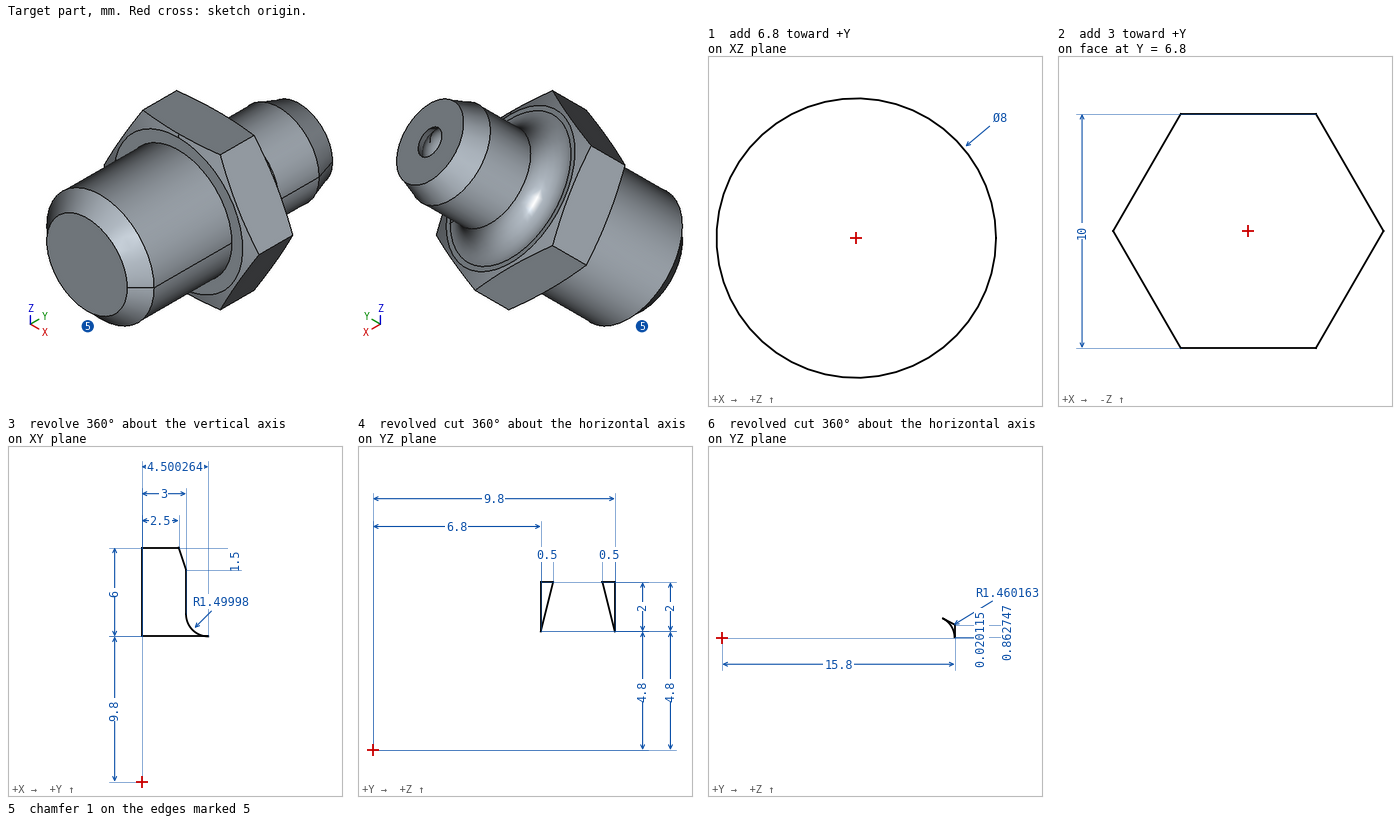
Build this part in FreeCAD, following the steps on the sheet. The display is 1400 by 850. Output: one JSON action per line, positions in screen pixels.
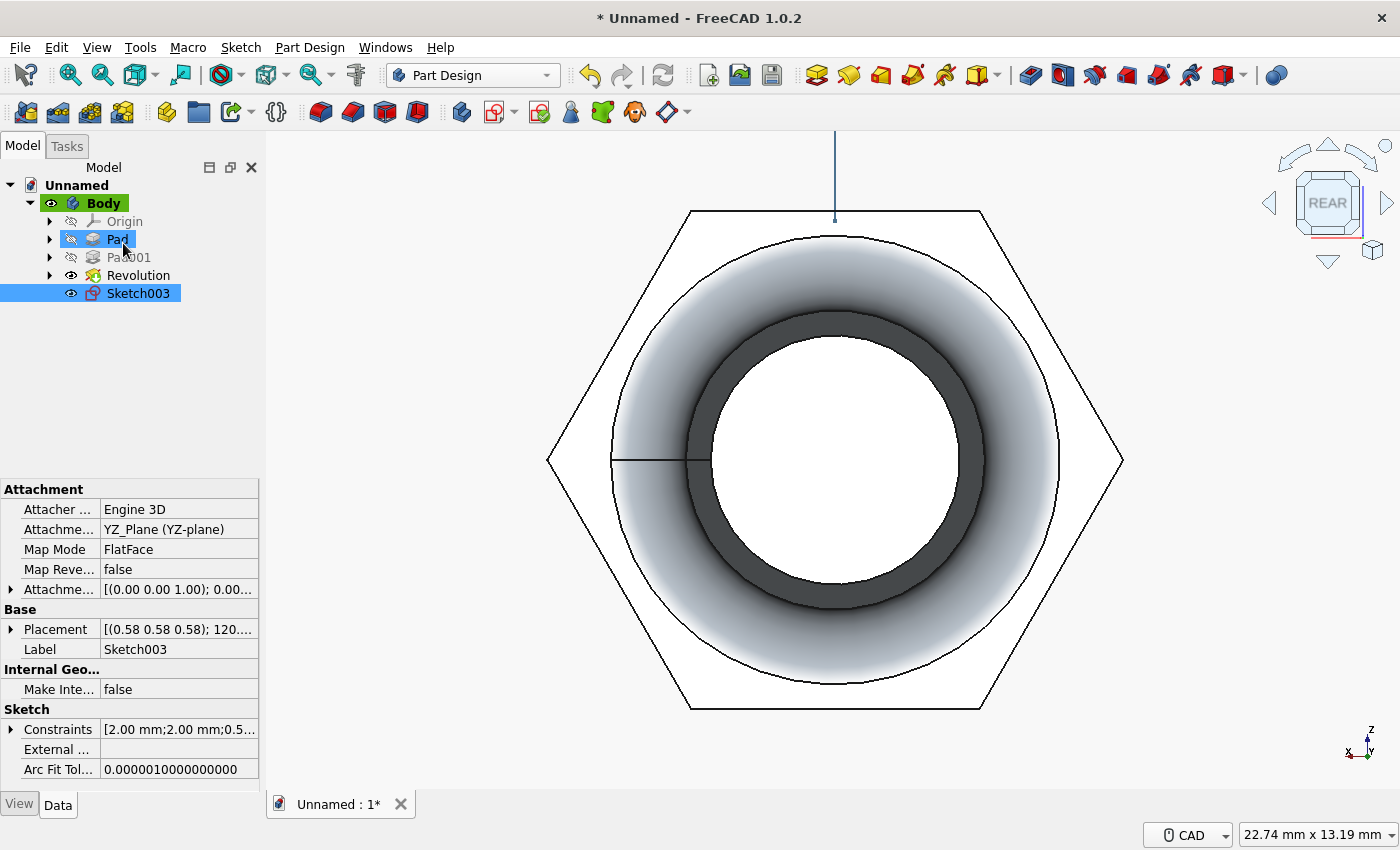
{"action": "left_click", "coordinate": [1096, 76]}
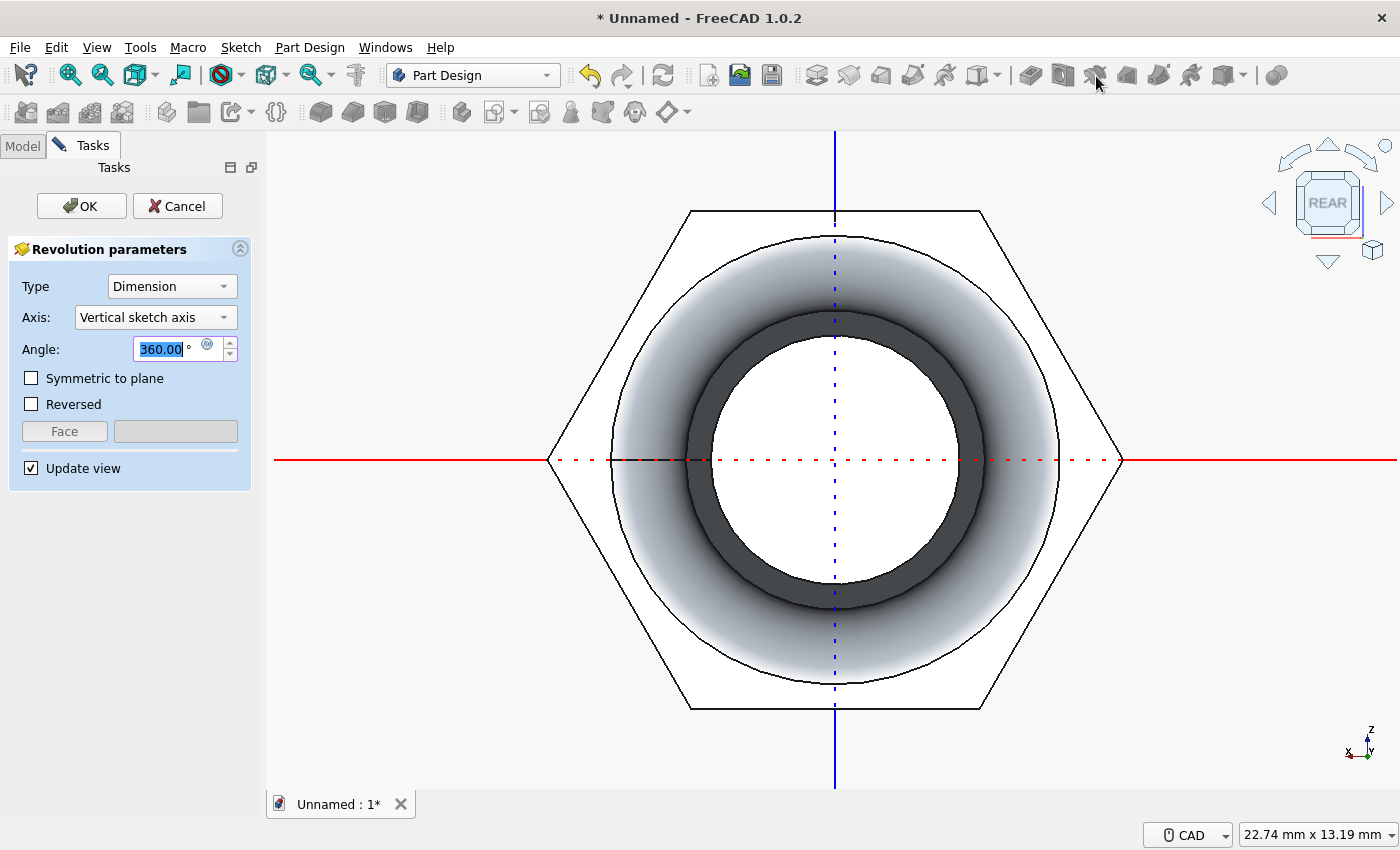
{"action": "left_click", "coordinate": [156, 318]}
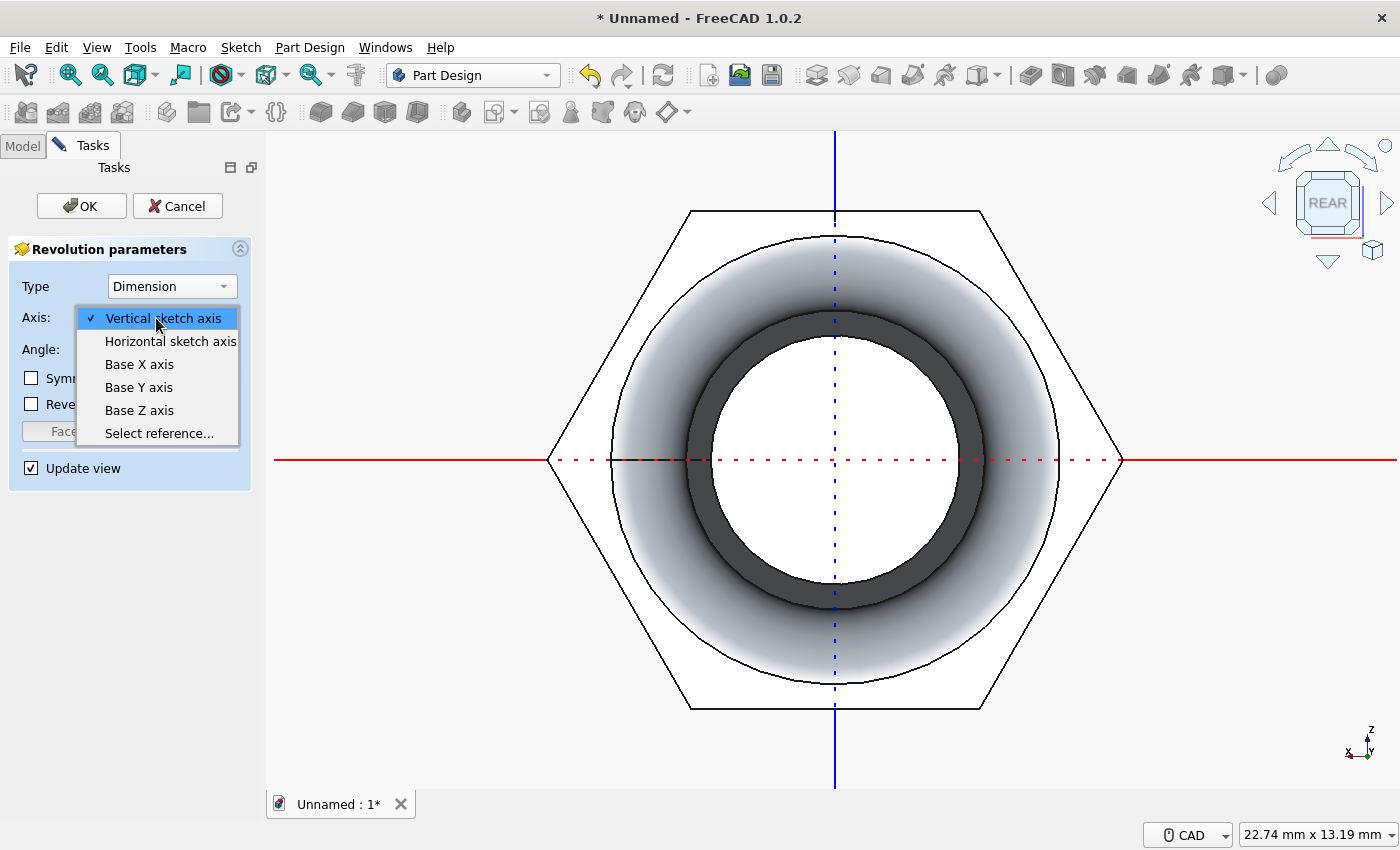
{"action": "left_click", "coordinate": [156, 342]}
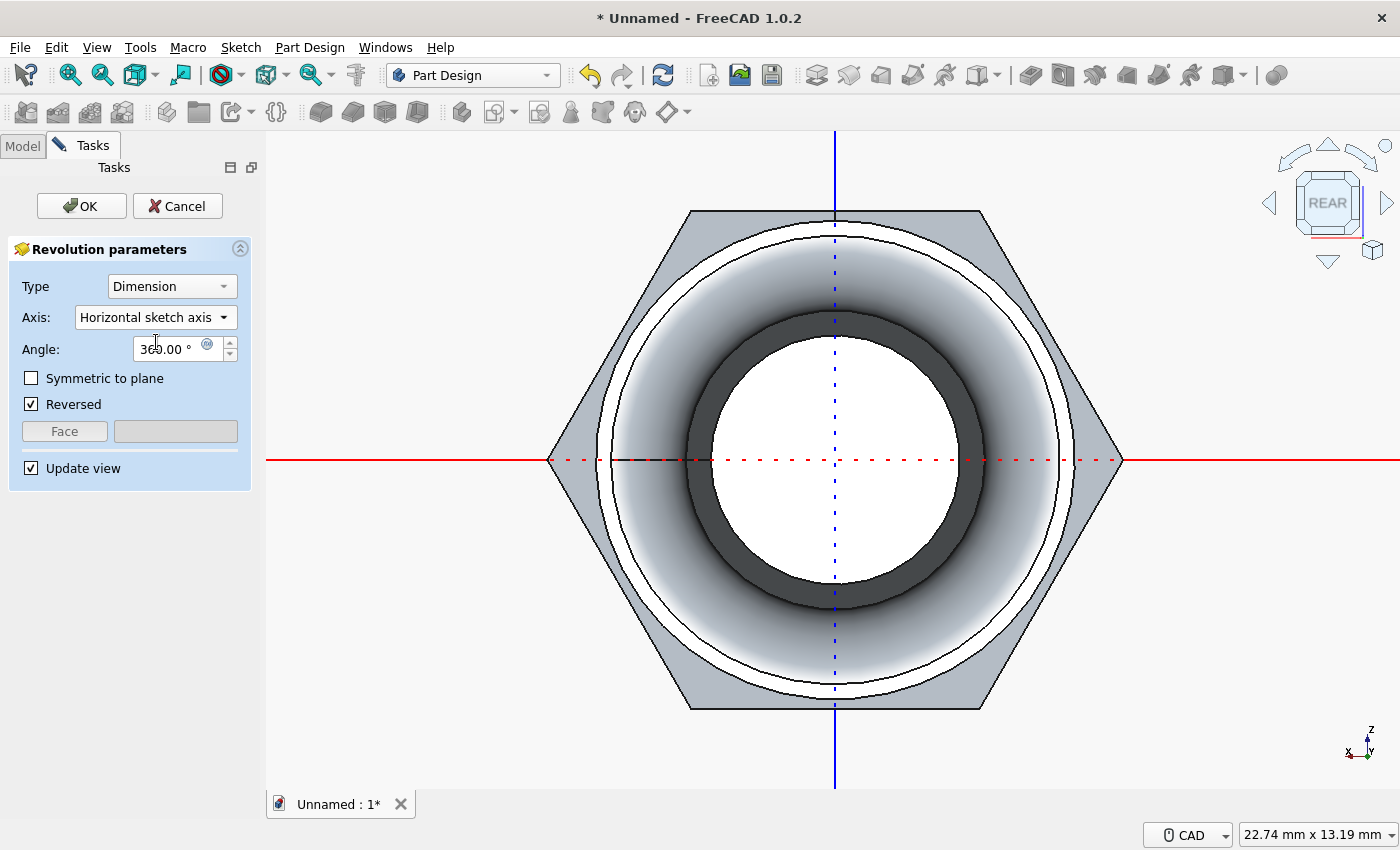
{"action": "left_click", "coordinate": [82, 206]}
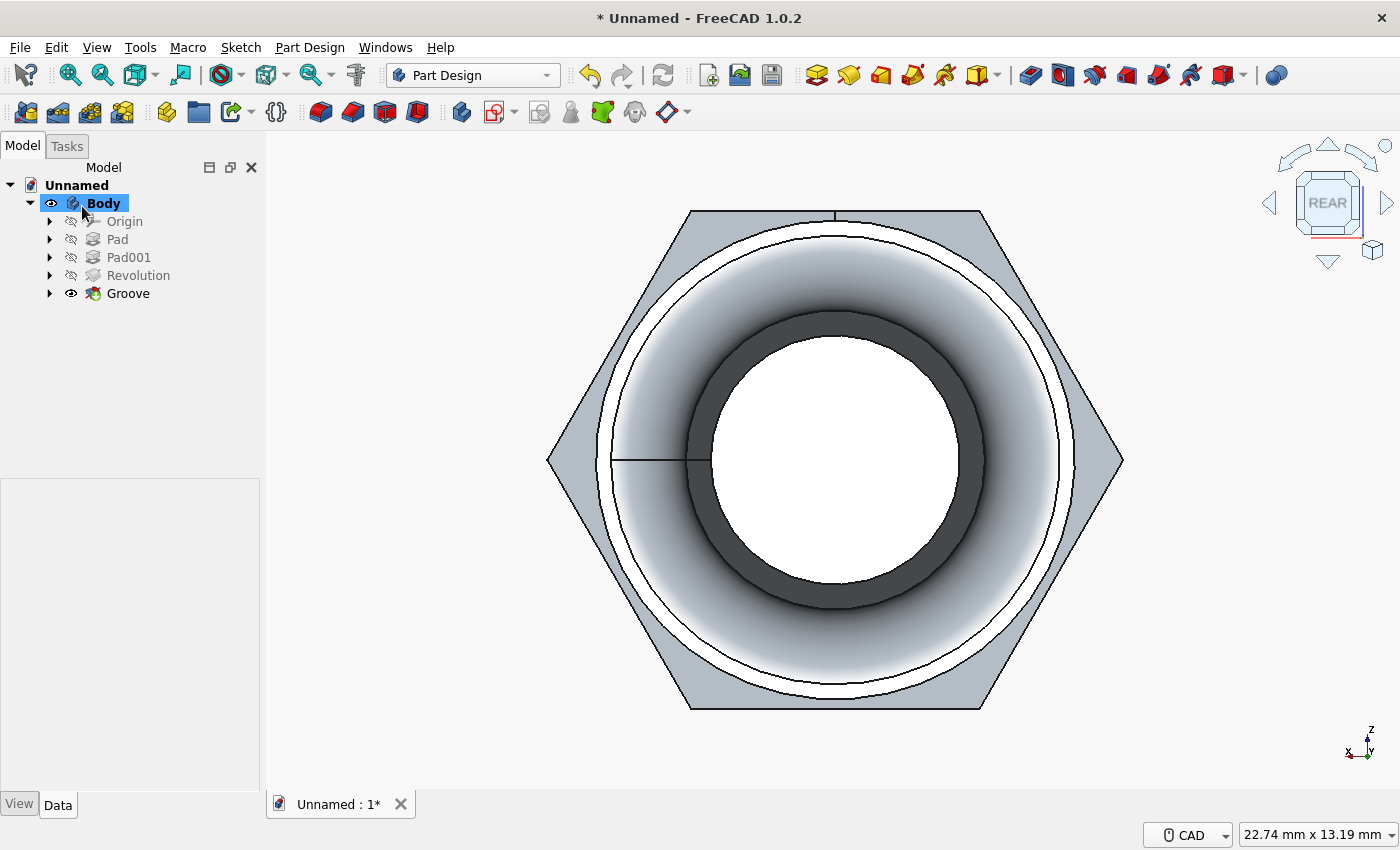
{"action": "key", "text": "0"}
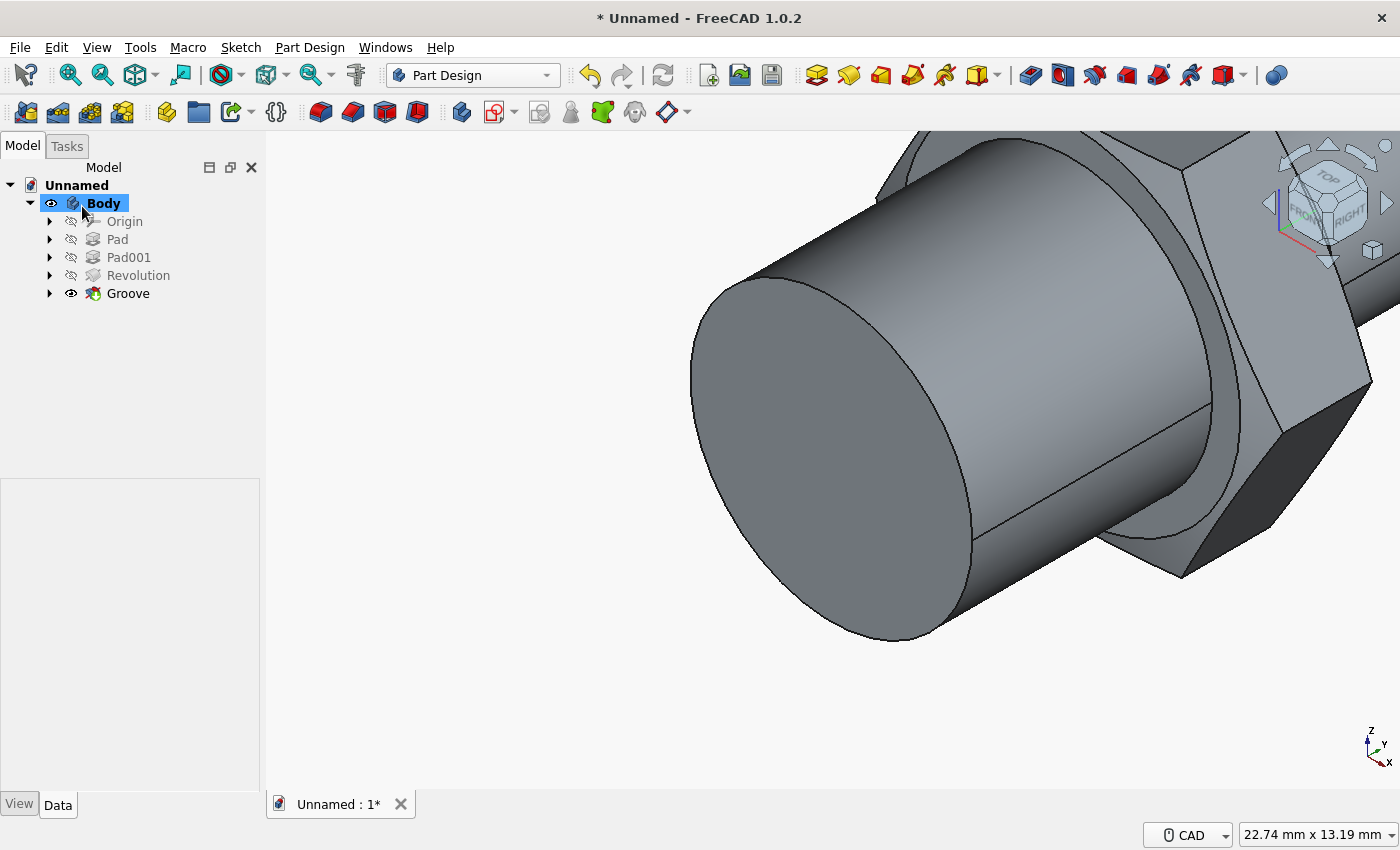
{"action": "left_click", "coordinate": [72, 76]}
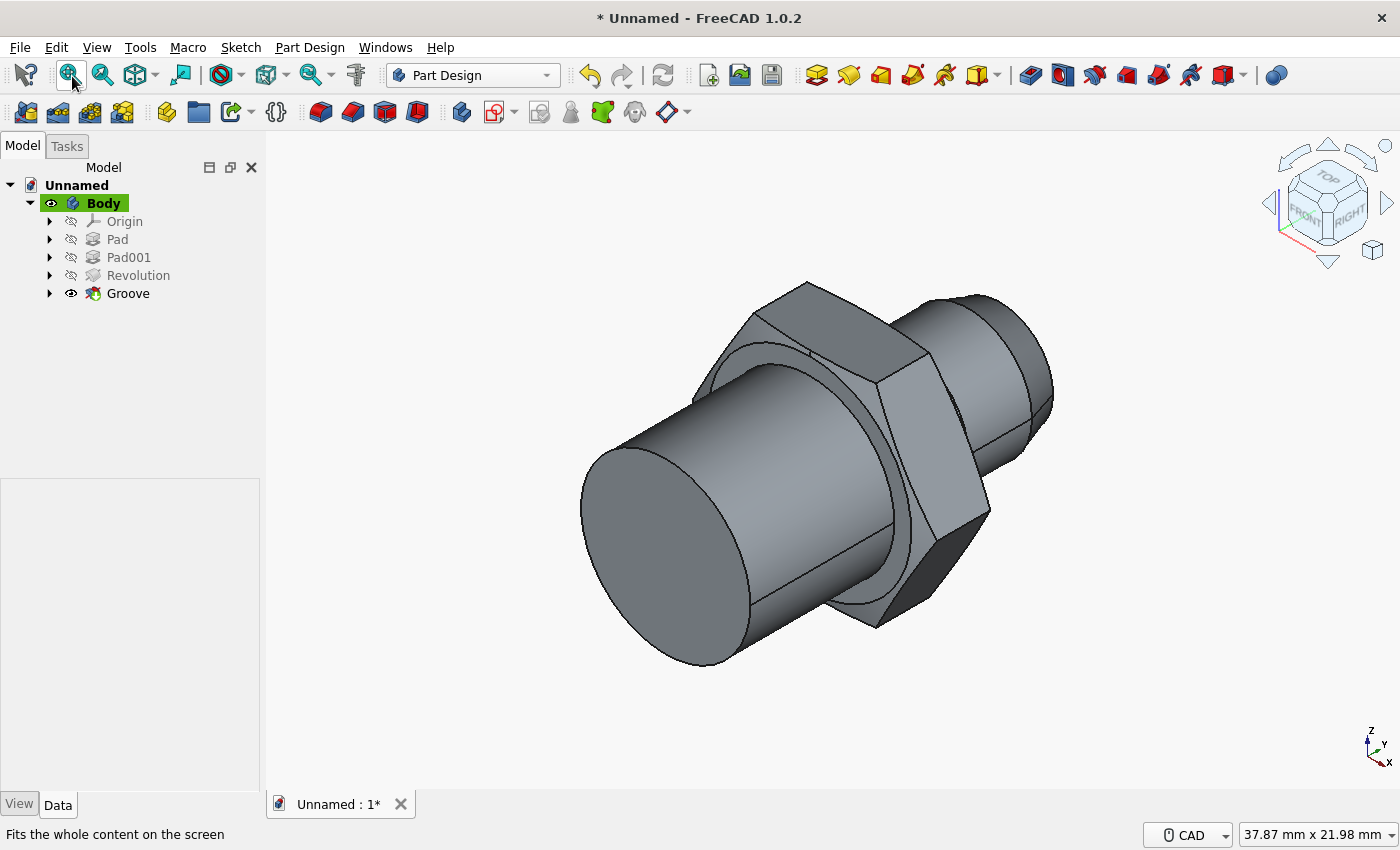
{"action": "left_click", "coordinate": [640, 447]}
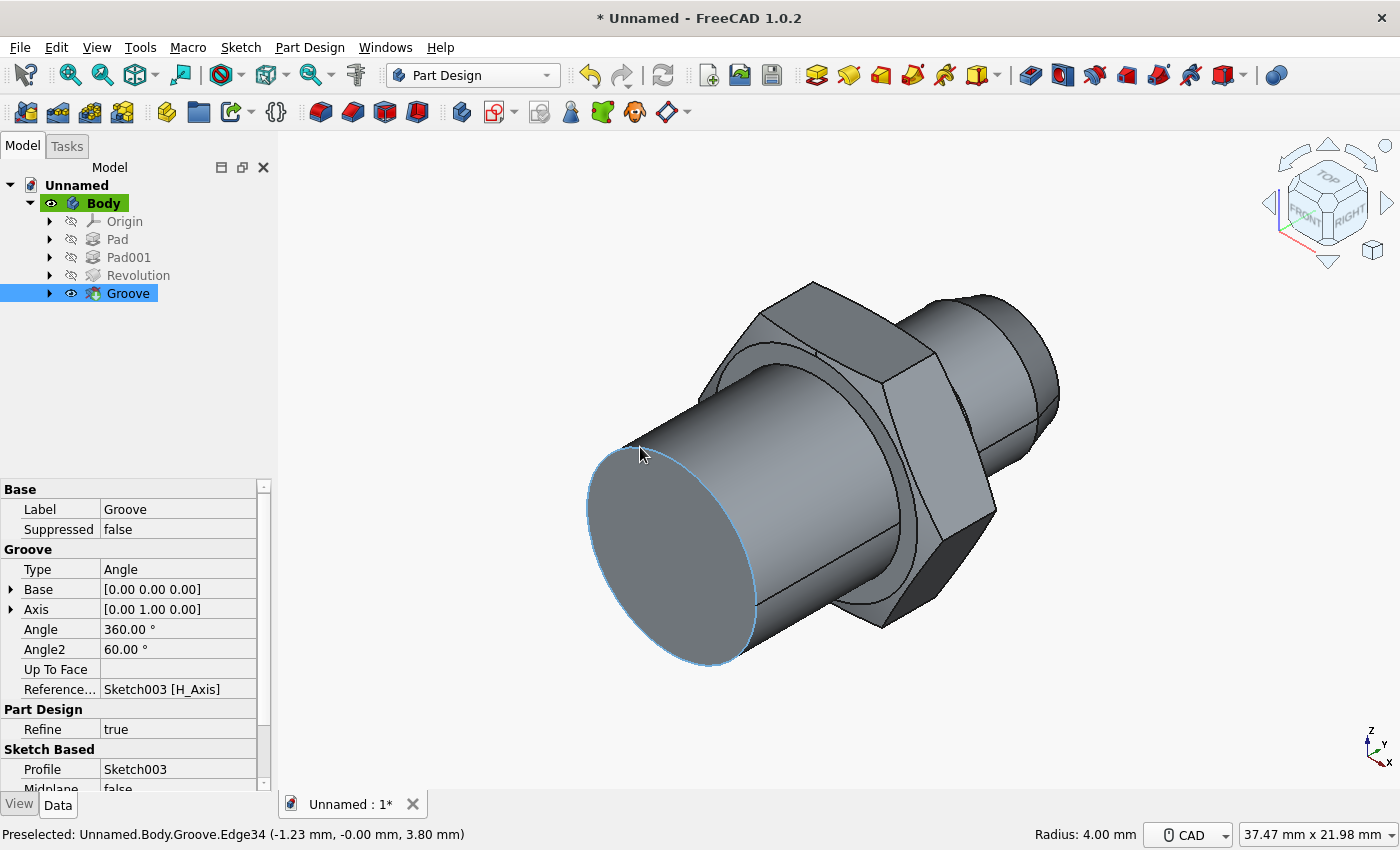
{"action": "left_click", "coordinate": [354, 112]}